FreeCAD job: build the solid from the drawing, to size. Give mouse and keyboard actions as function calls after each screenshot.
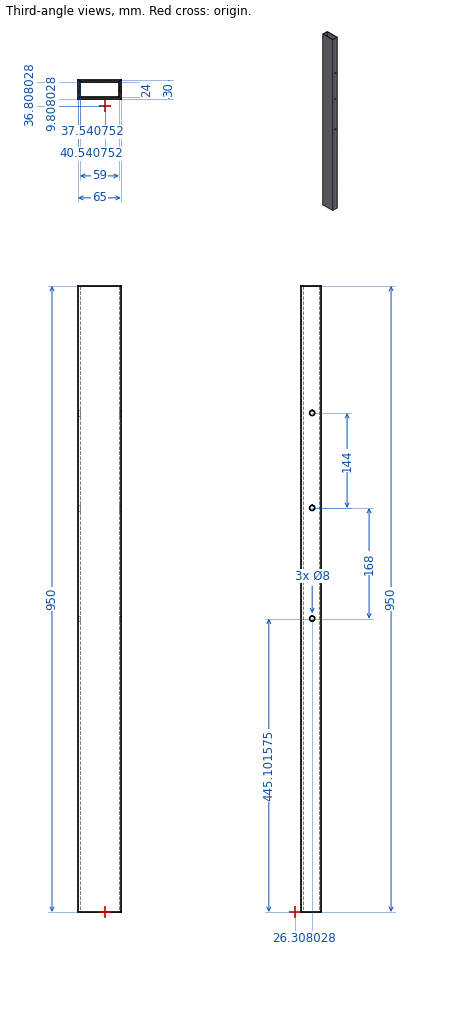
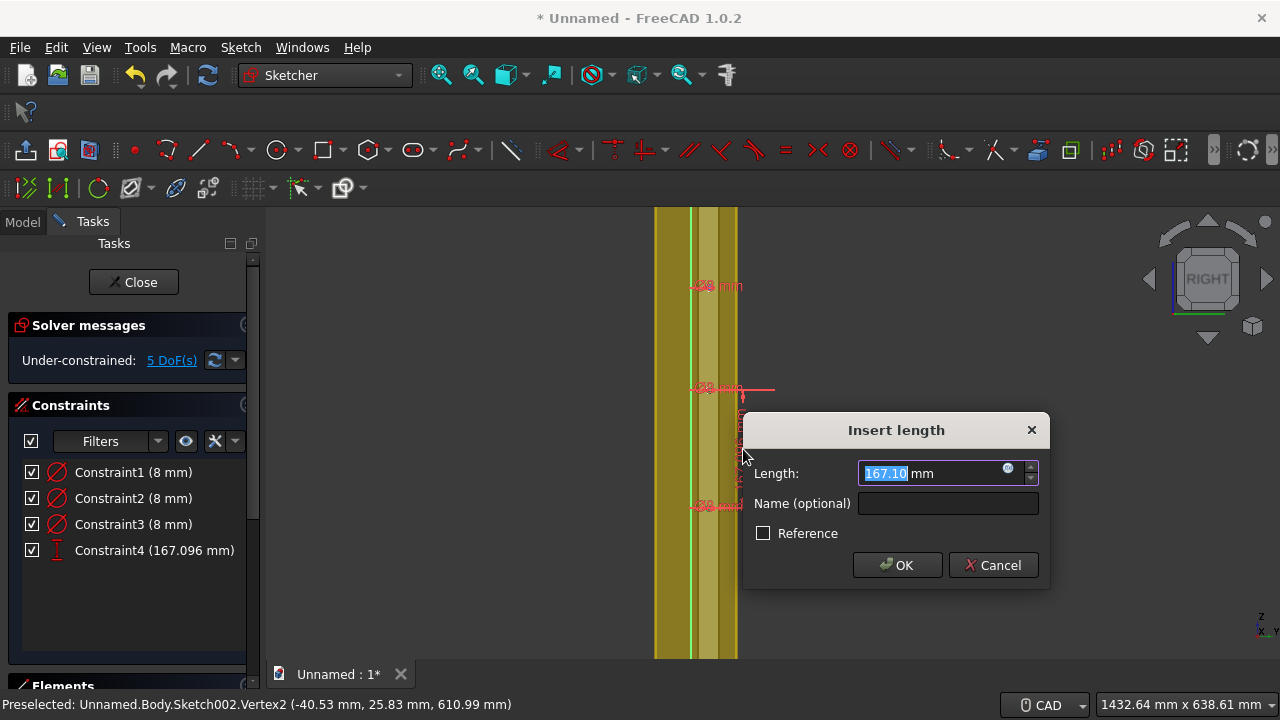
text(168)
key(Return)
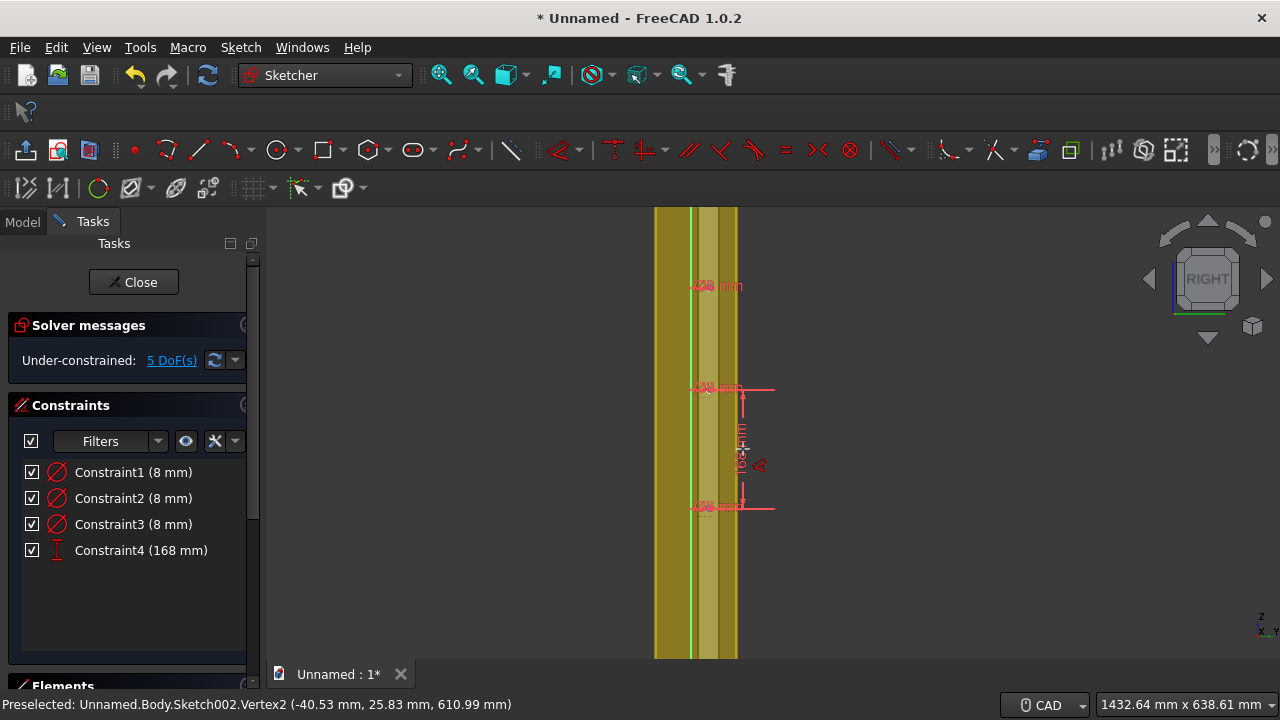
click(709, 390)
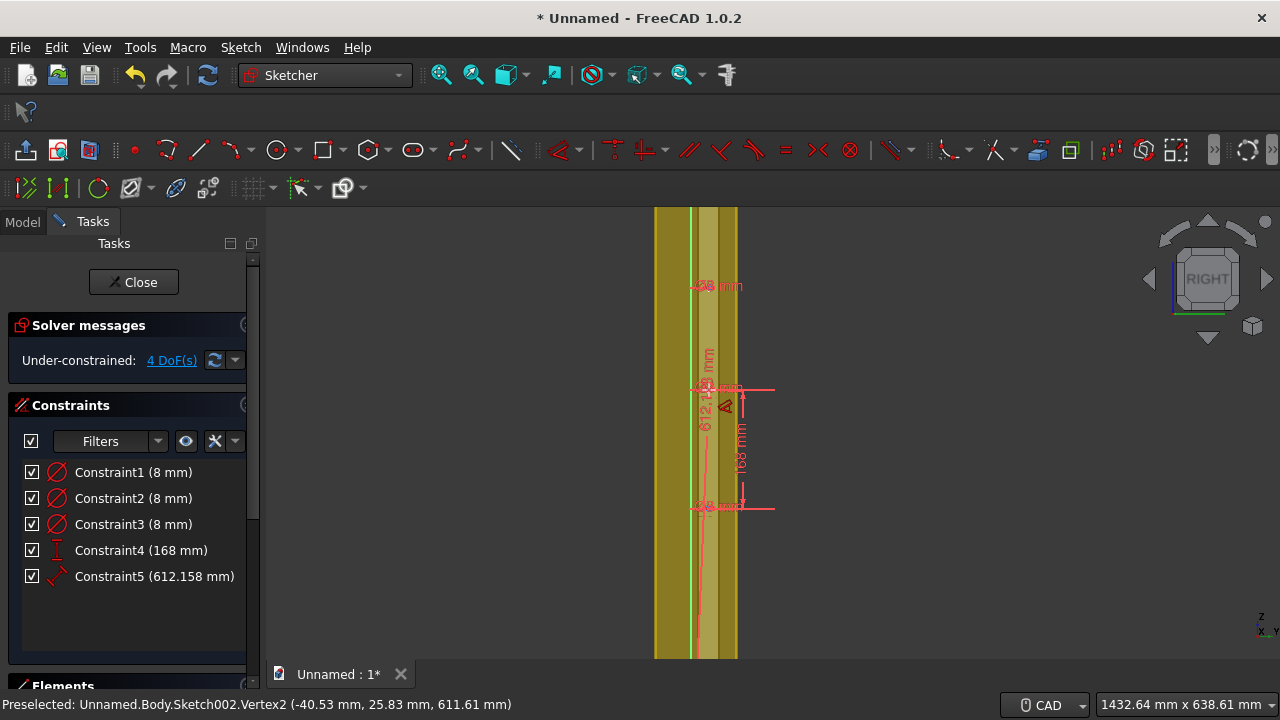
click(709, 288)
click(743, 339)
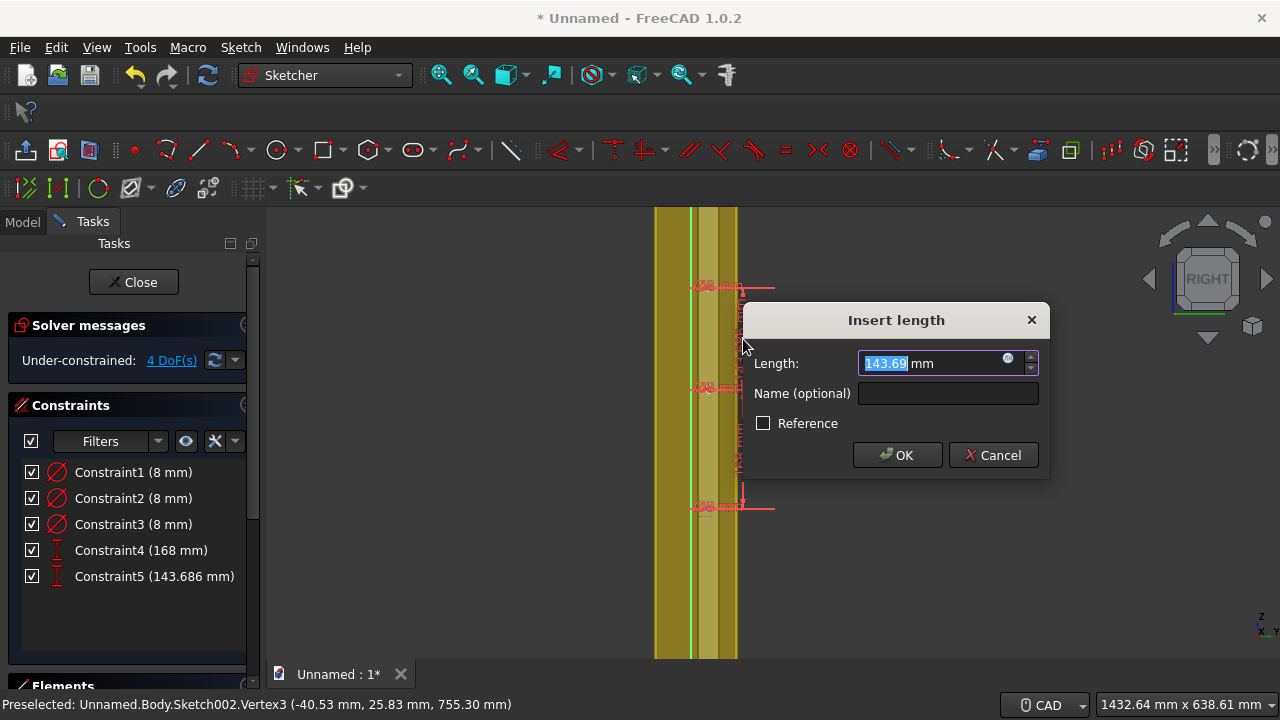
text(144)
key(Return)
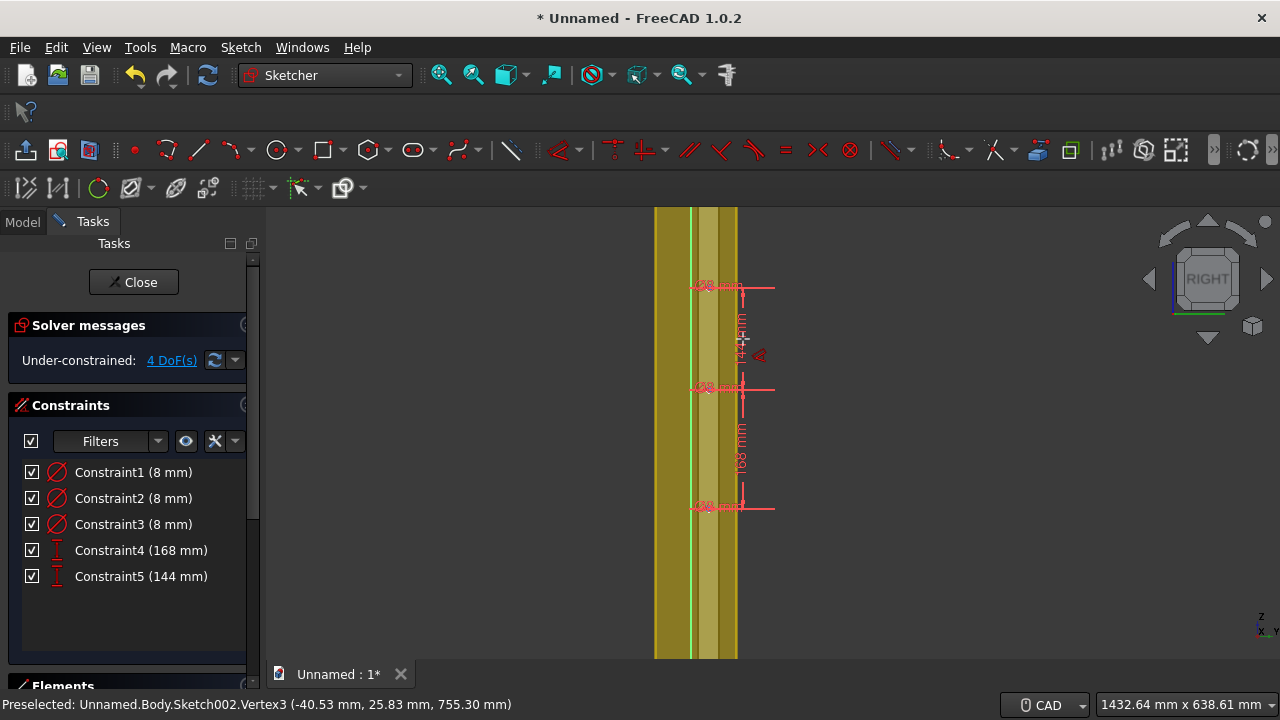
scroll(709, 509, up, 4)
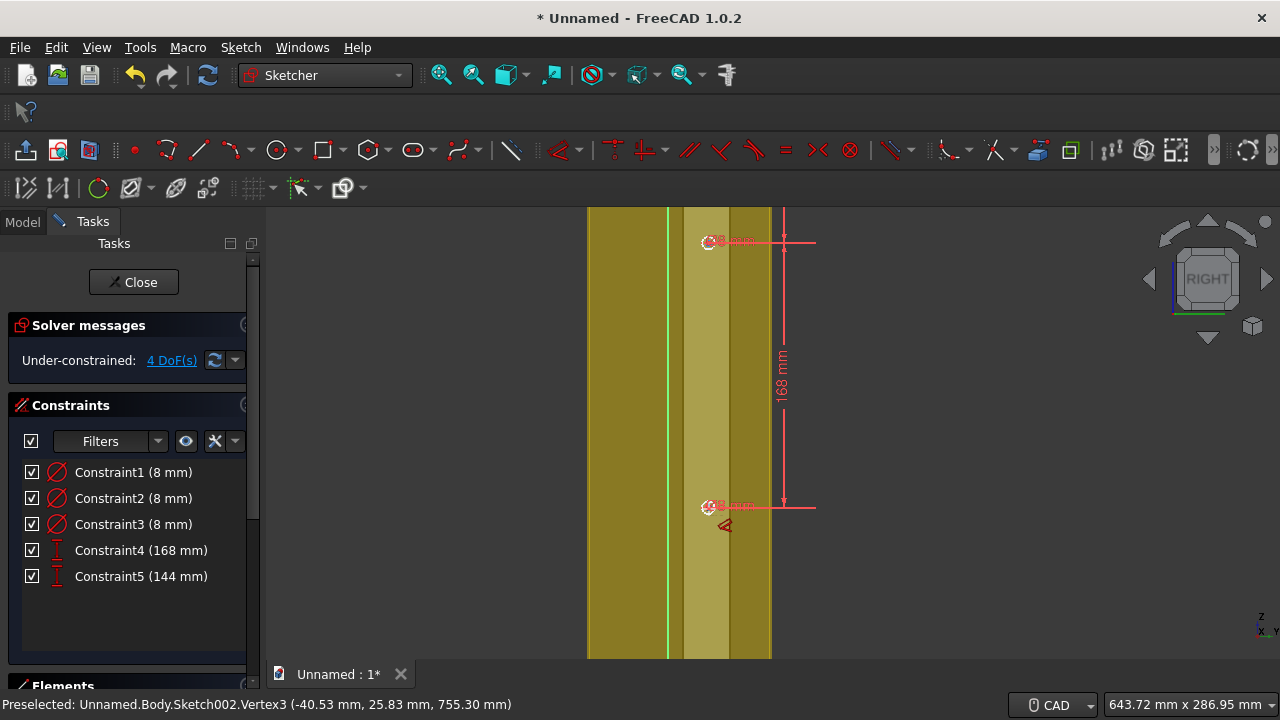
click(708, 508)
click(688, 474)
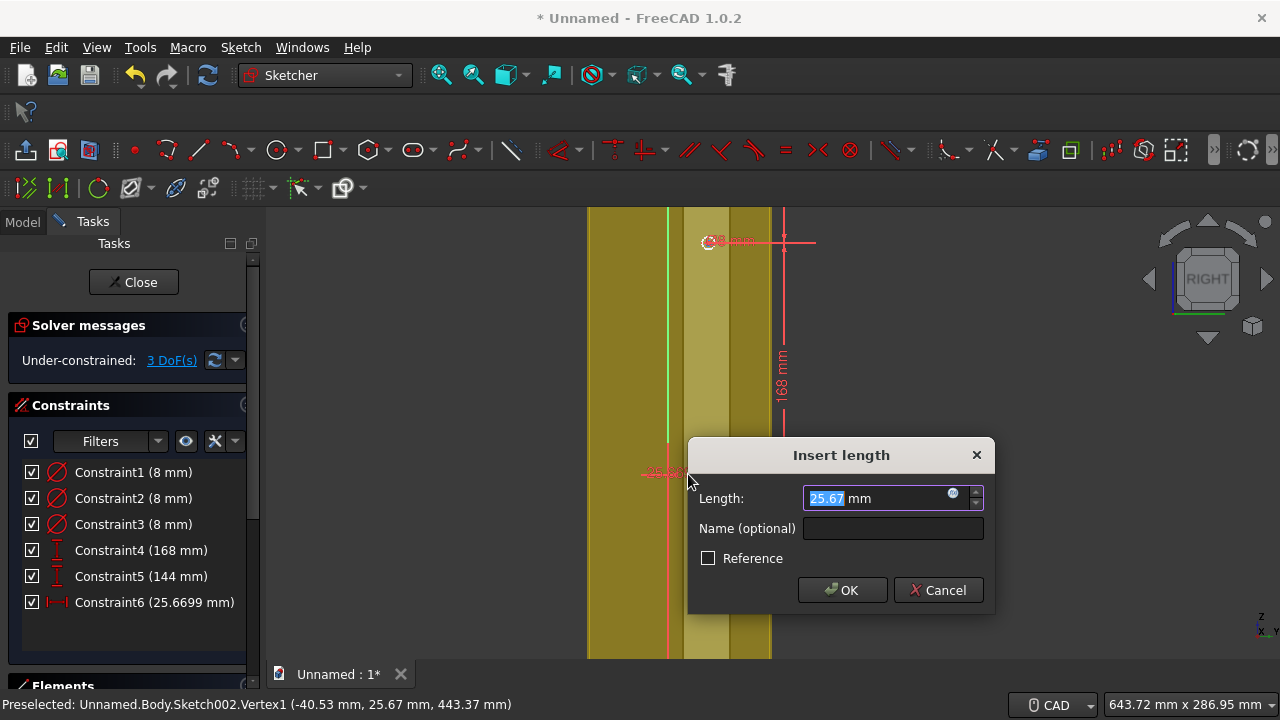
text(26.308028)
key(Return)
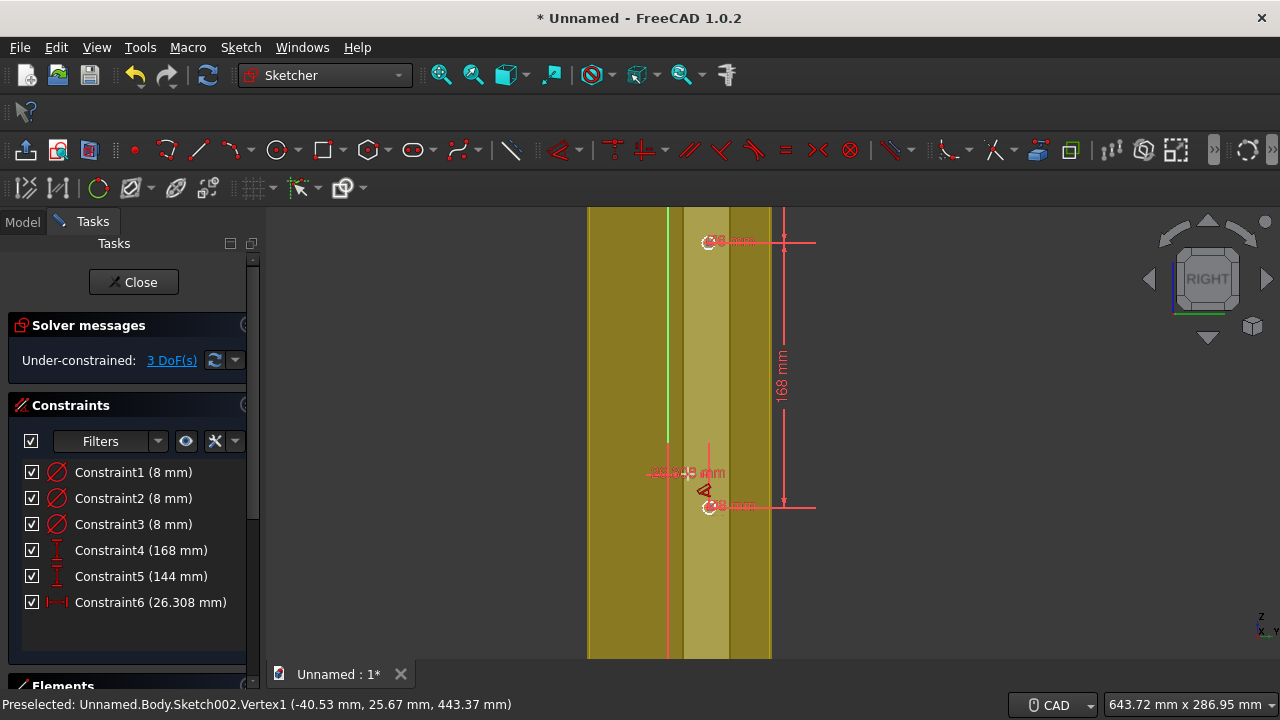
click(708, 243)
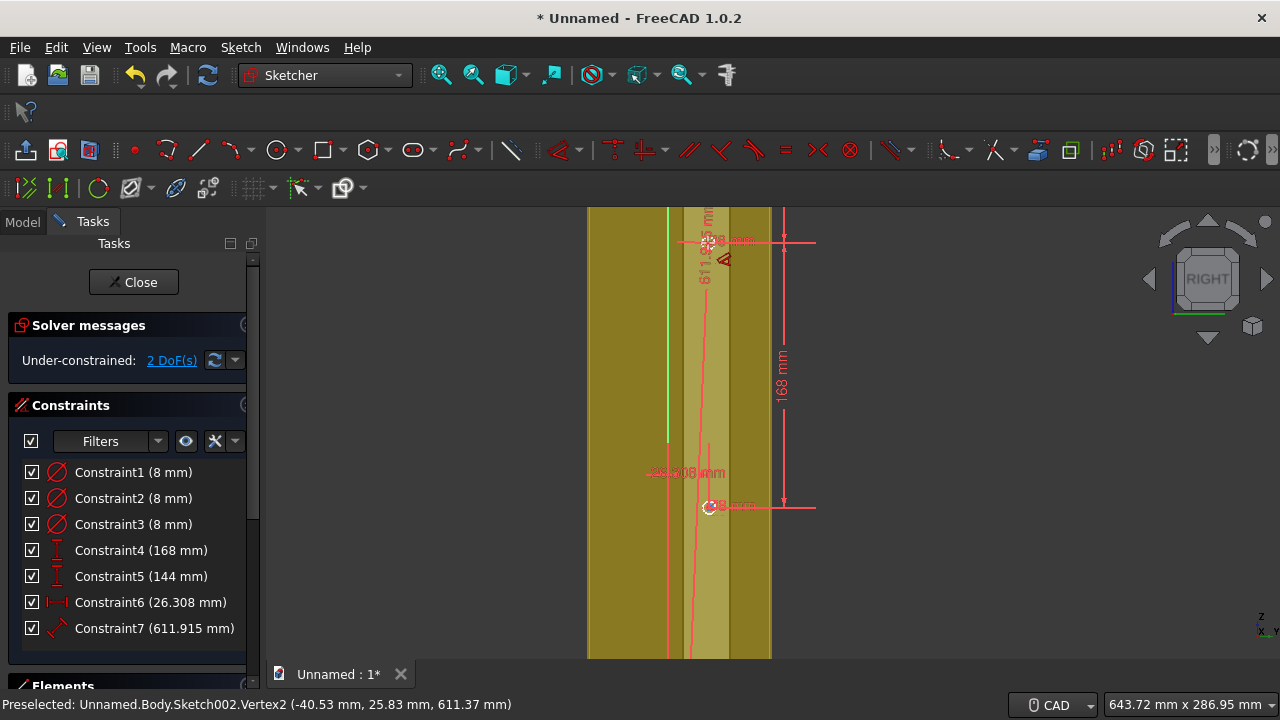
key(Escape)
key(Escape)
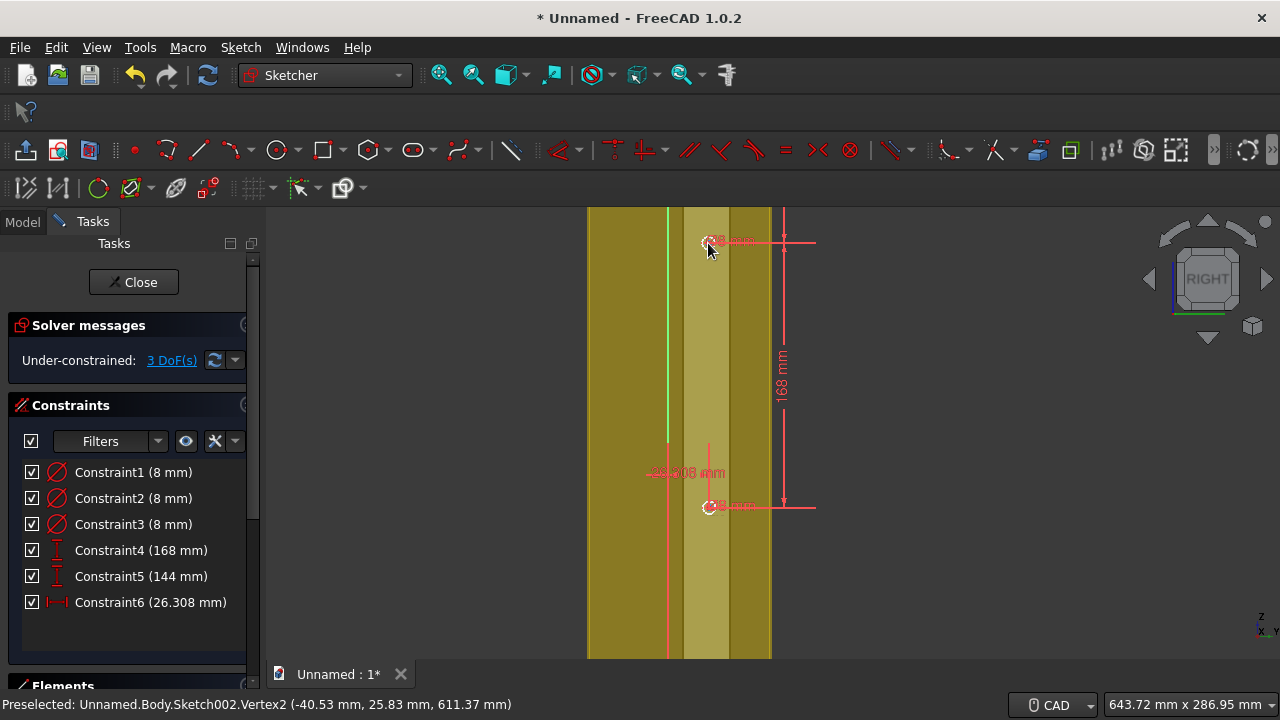
click(708, 243)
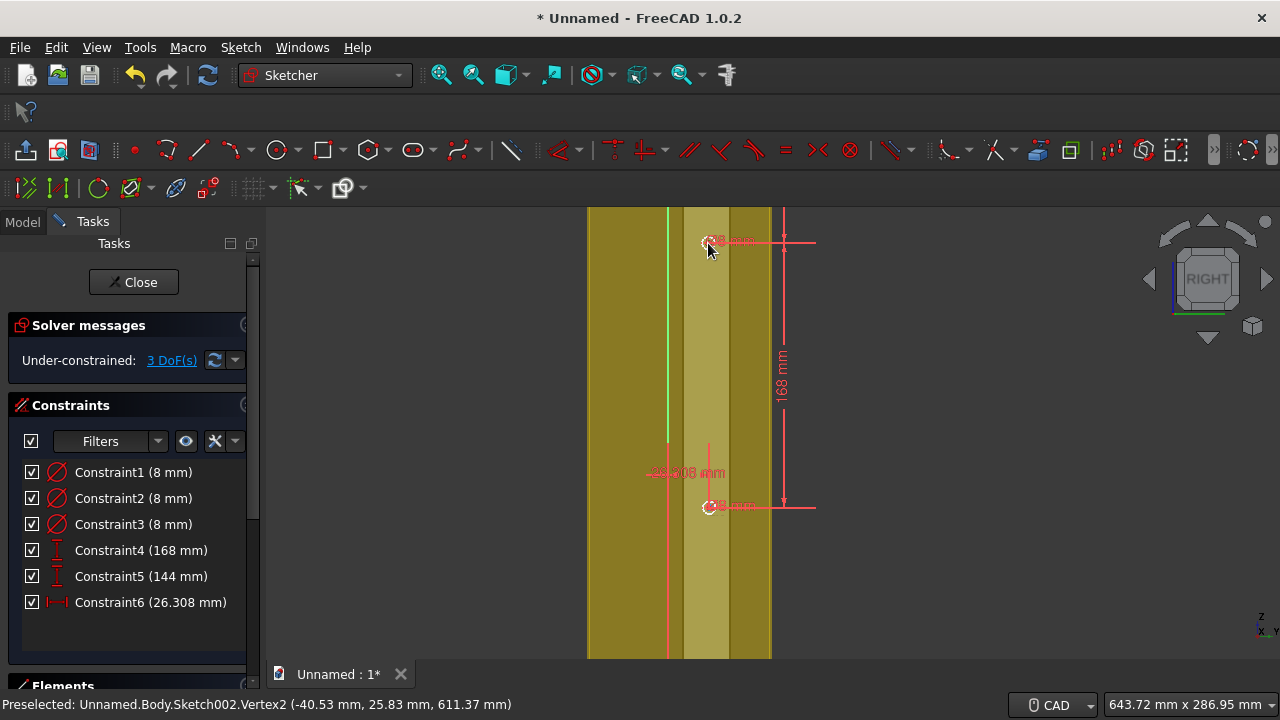
click(582, 150)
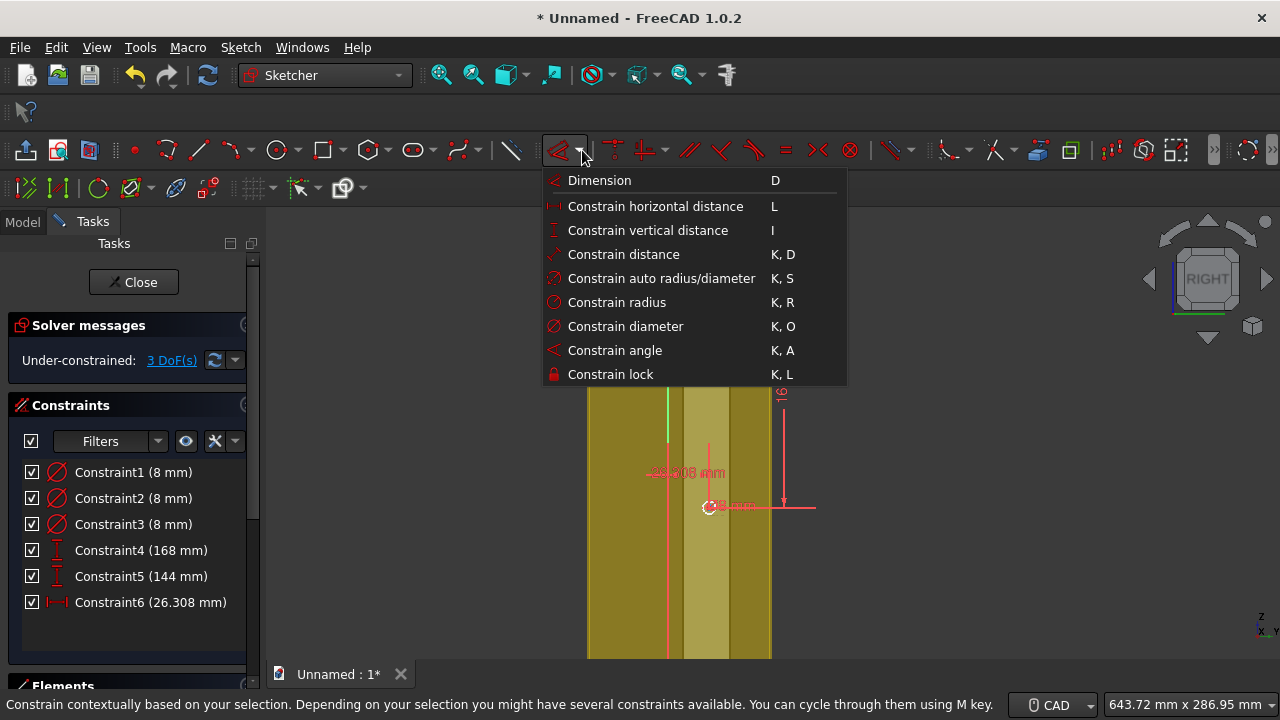
click(695, 206)